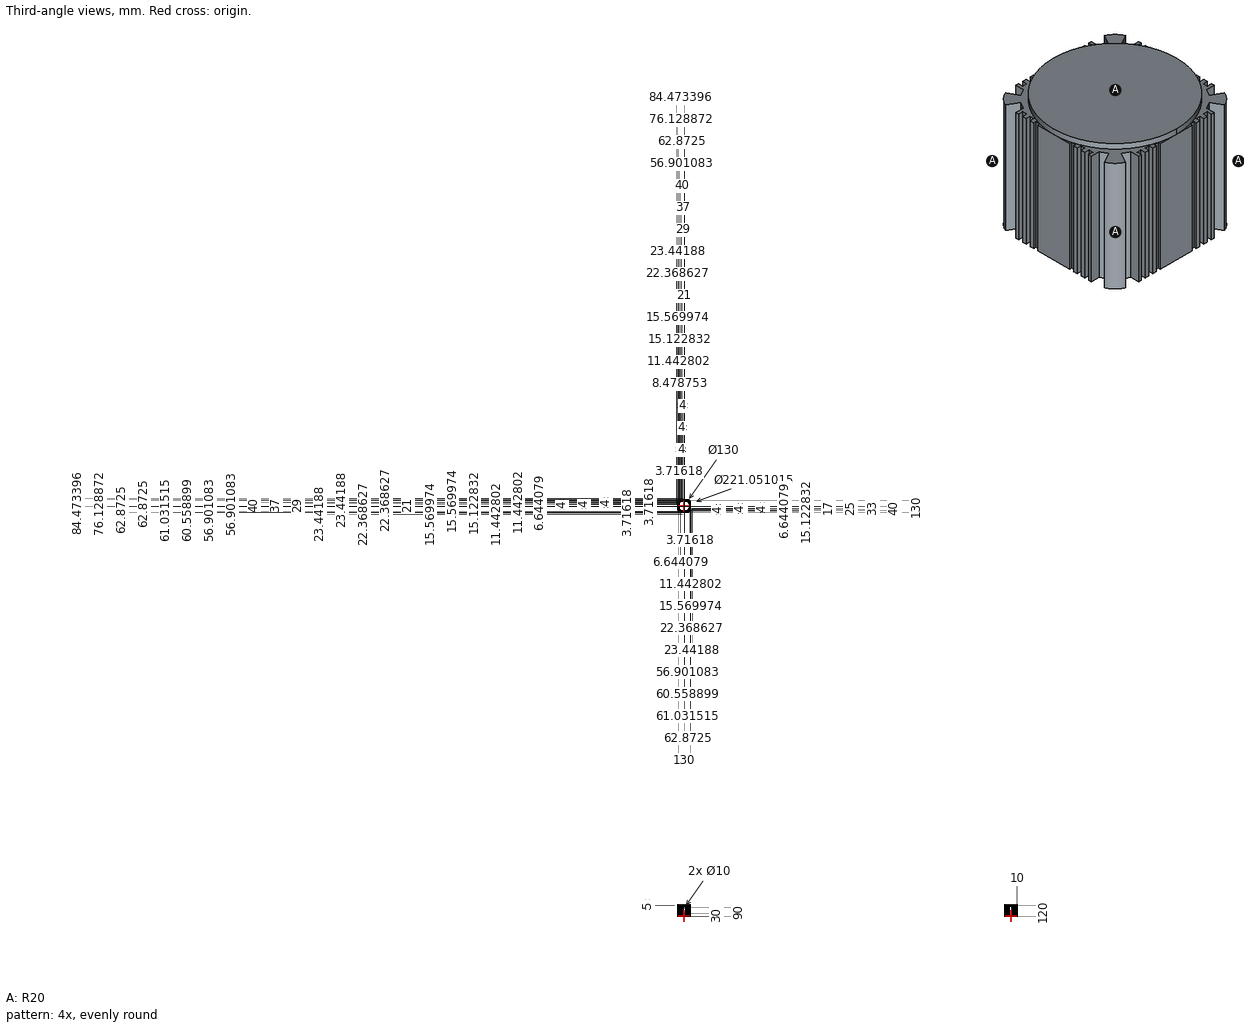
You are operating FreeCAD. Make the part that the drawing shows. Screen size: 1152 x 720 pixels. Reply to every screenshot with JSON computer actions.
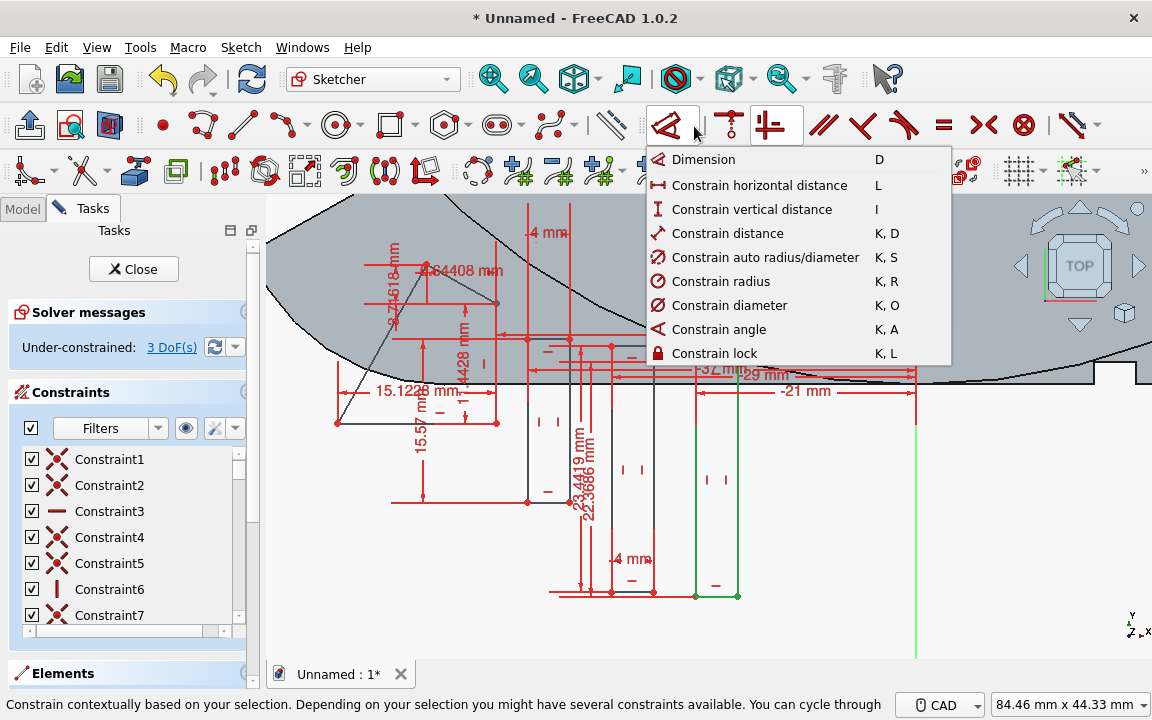
{"action": "left_click", "coordinate": [799, 209]}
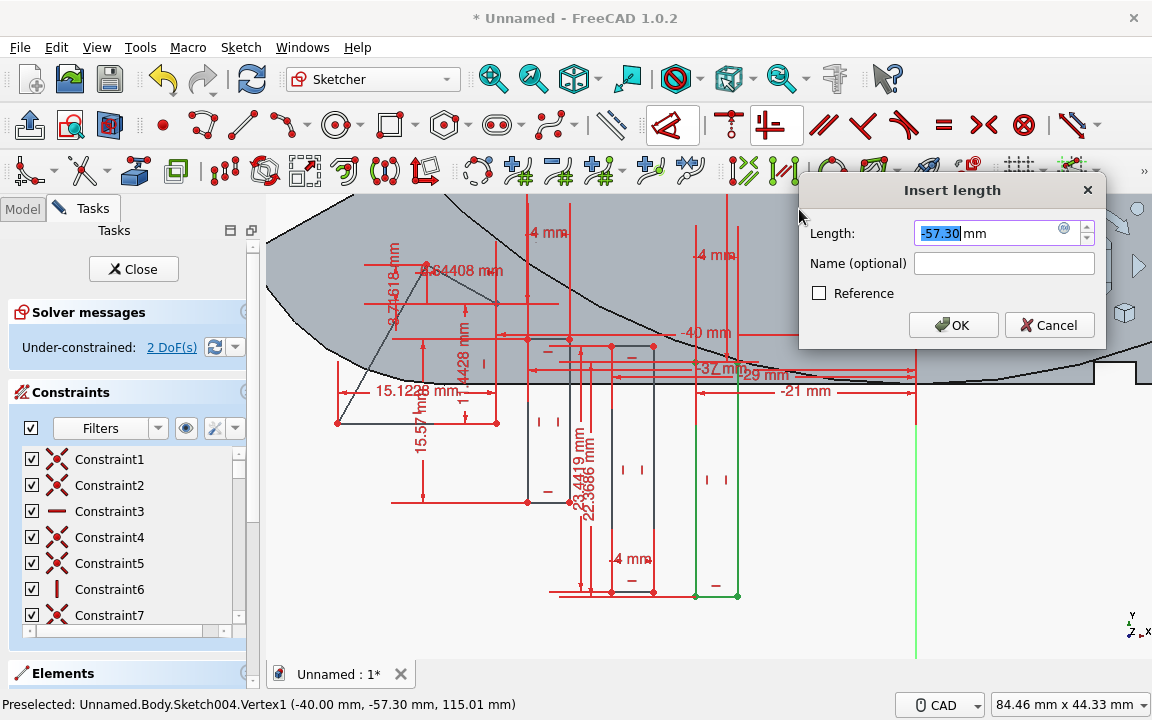
{"action": "type", "text": "-56.901083"}
{"action": "key", "text": "Return"}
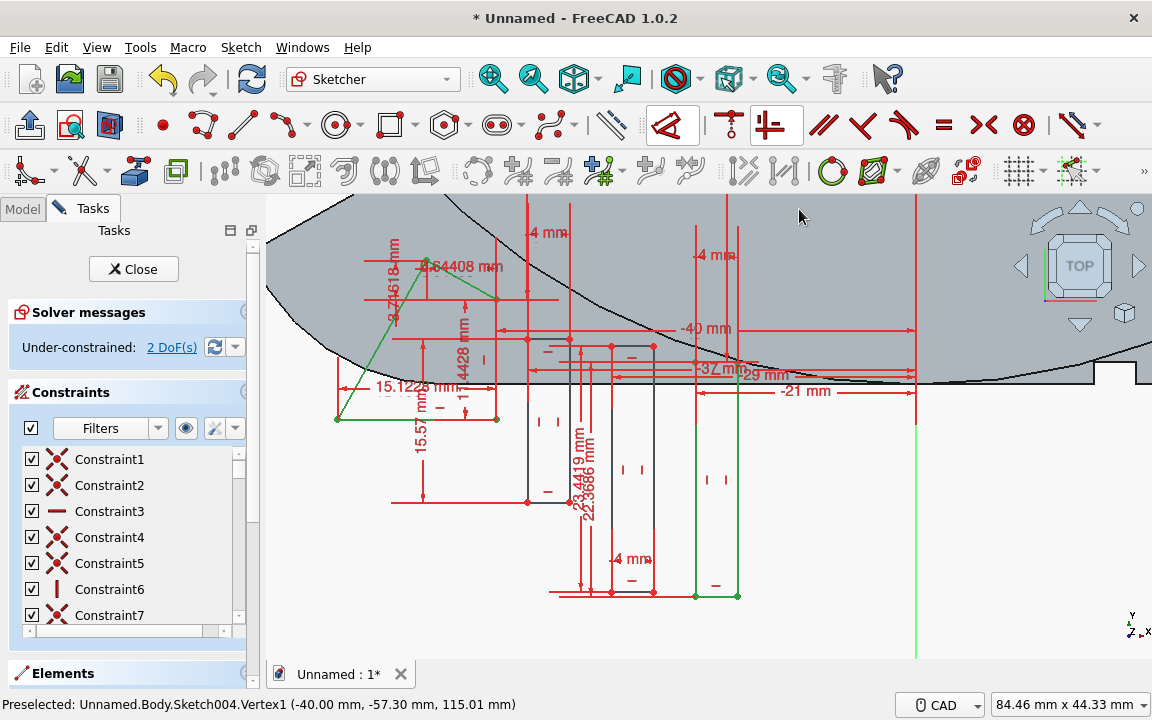
{"action": "left_click", "coordinate": [528, 339]}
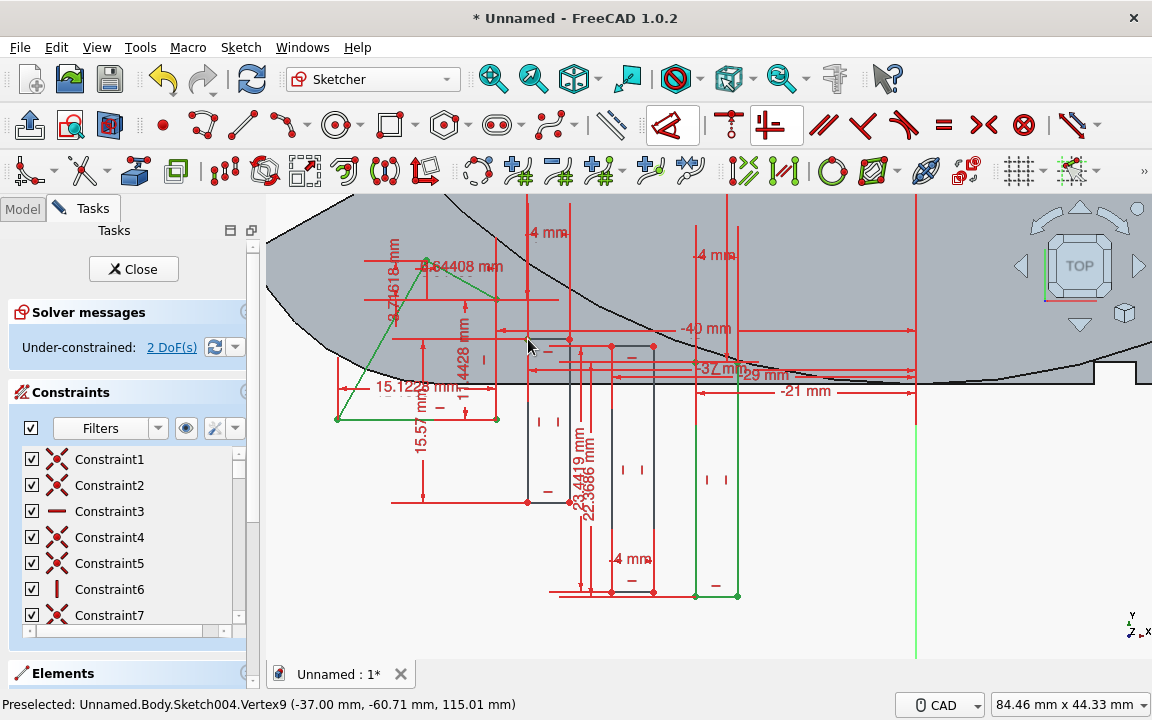
{"action": "left_click", "coordinate": [694, 126]}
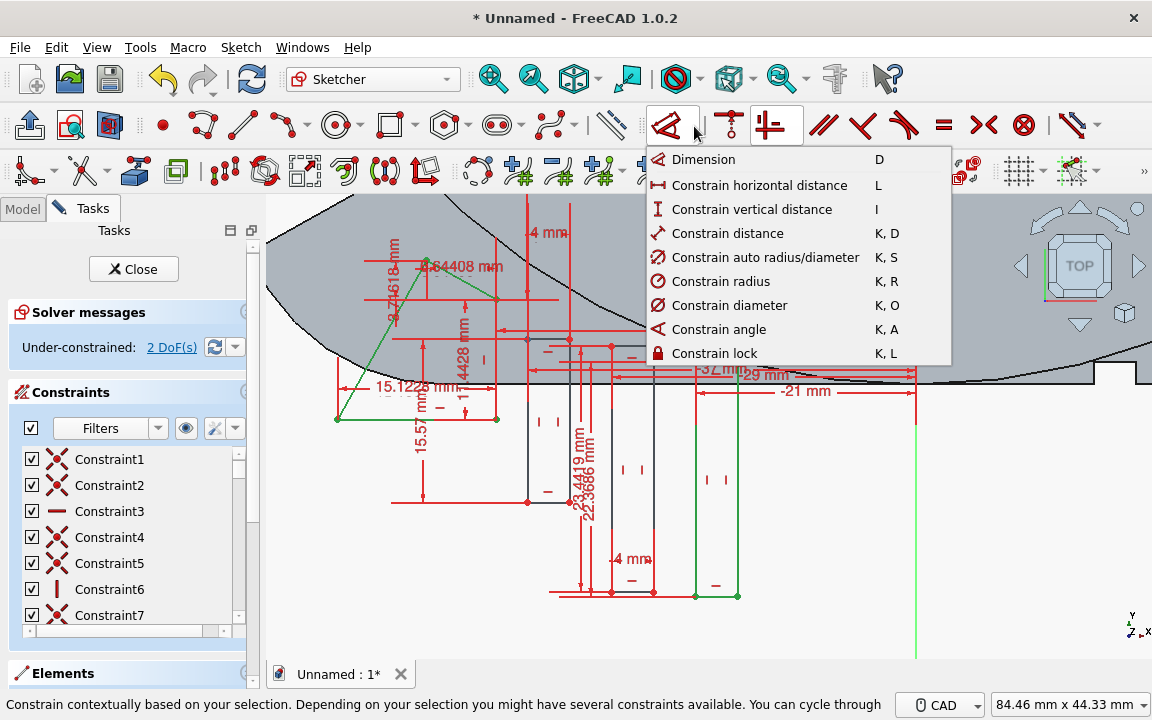
{"action": "left_click", "coordinate": [799, 209]}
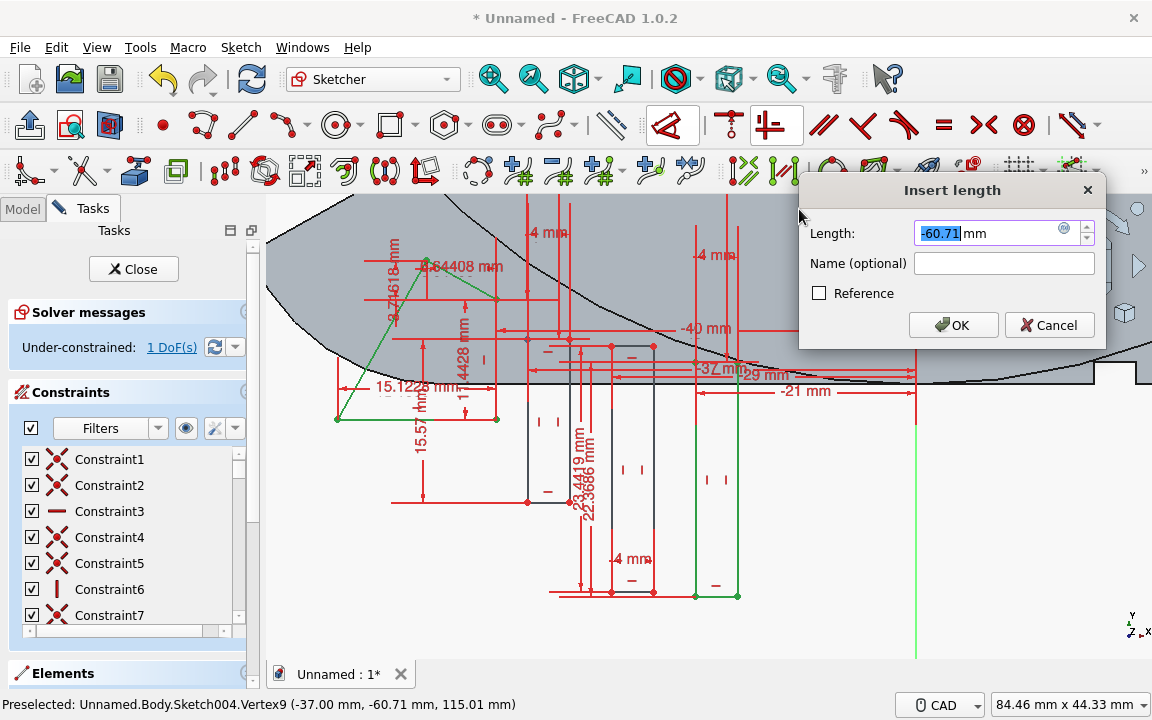
{"action": "type", "text": "-60.558899"}
{"action": "key", "text": "Return"}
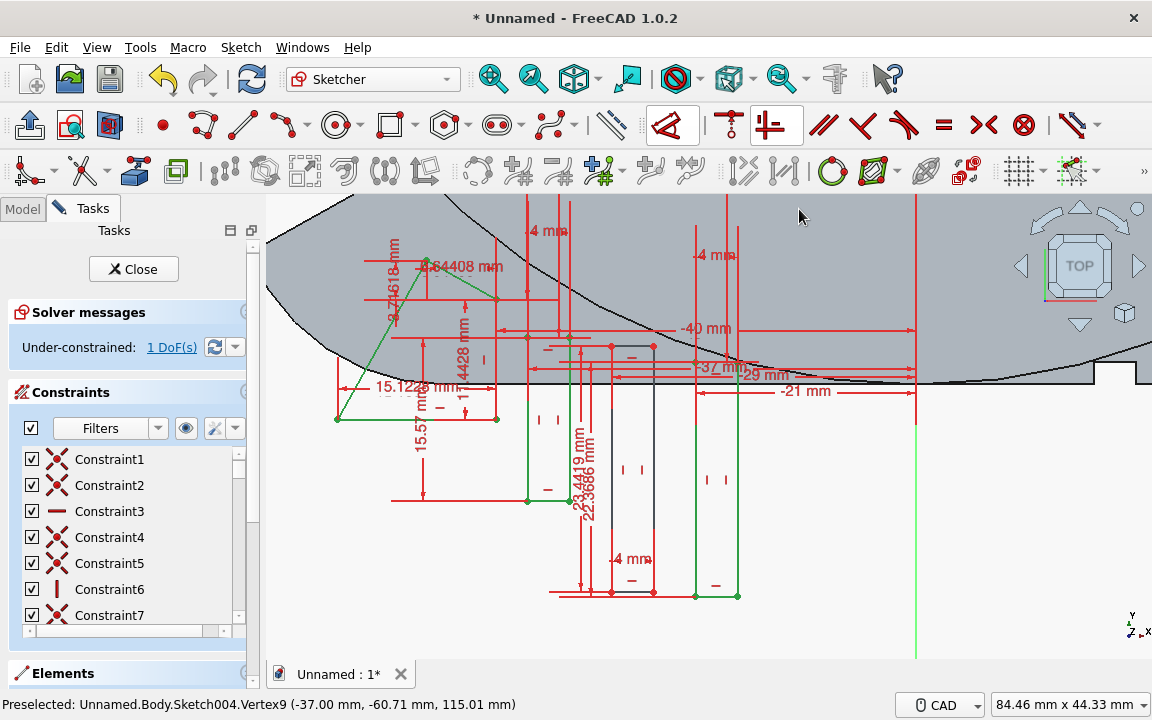
{"action": "left_click", "coordinate": [612, 346]}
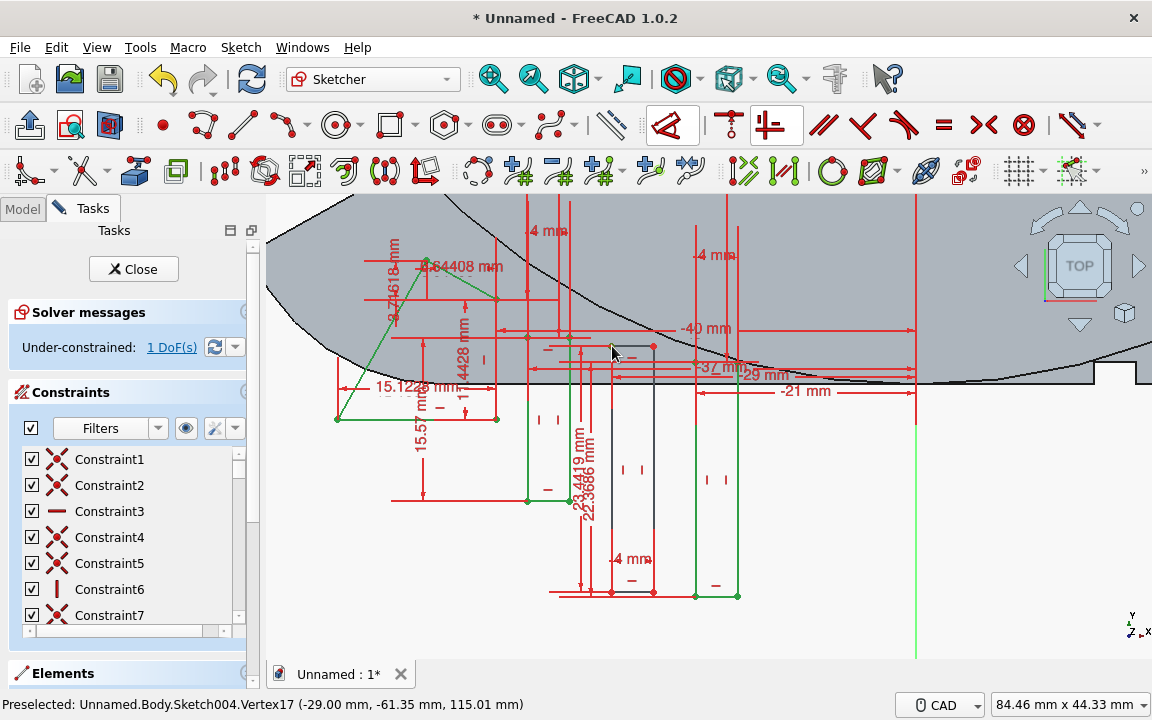
{"action": "left_click", "coordinate": [694, 126]}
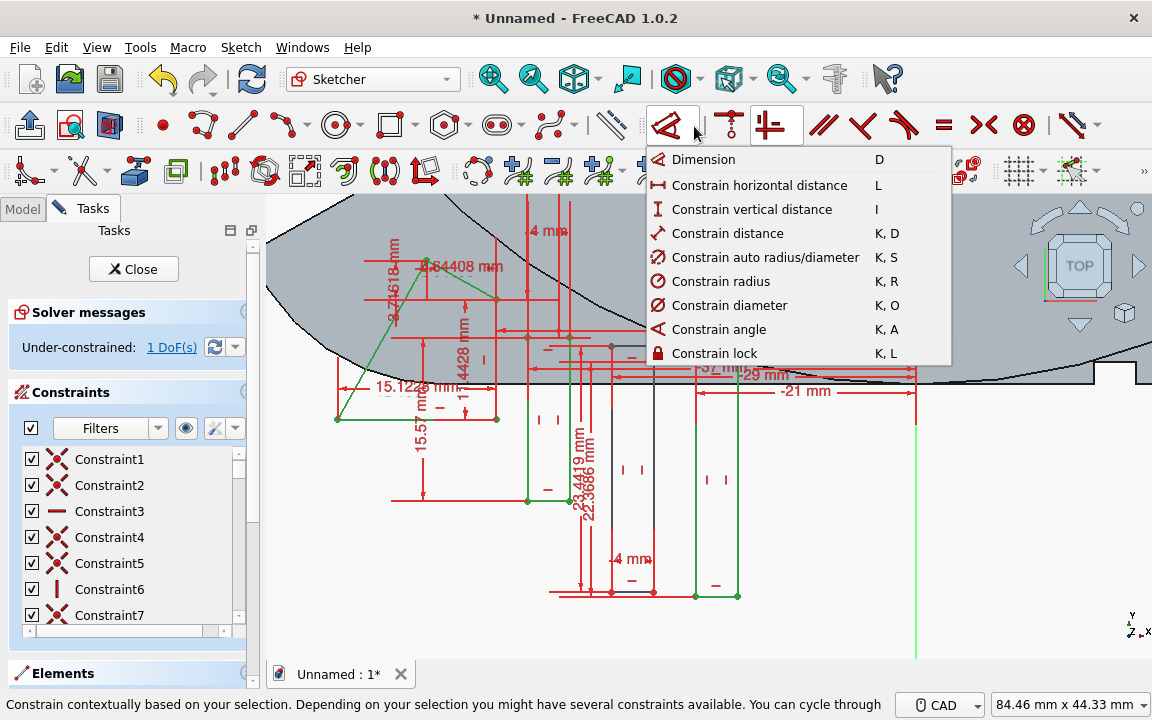
{"action": "left_click", "coordinate": [799, 209]}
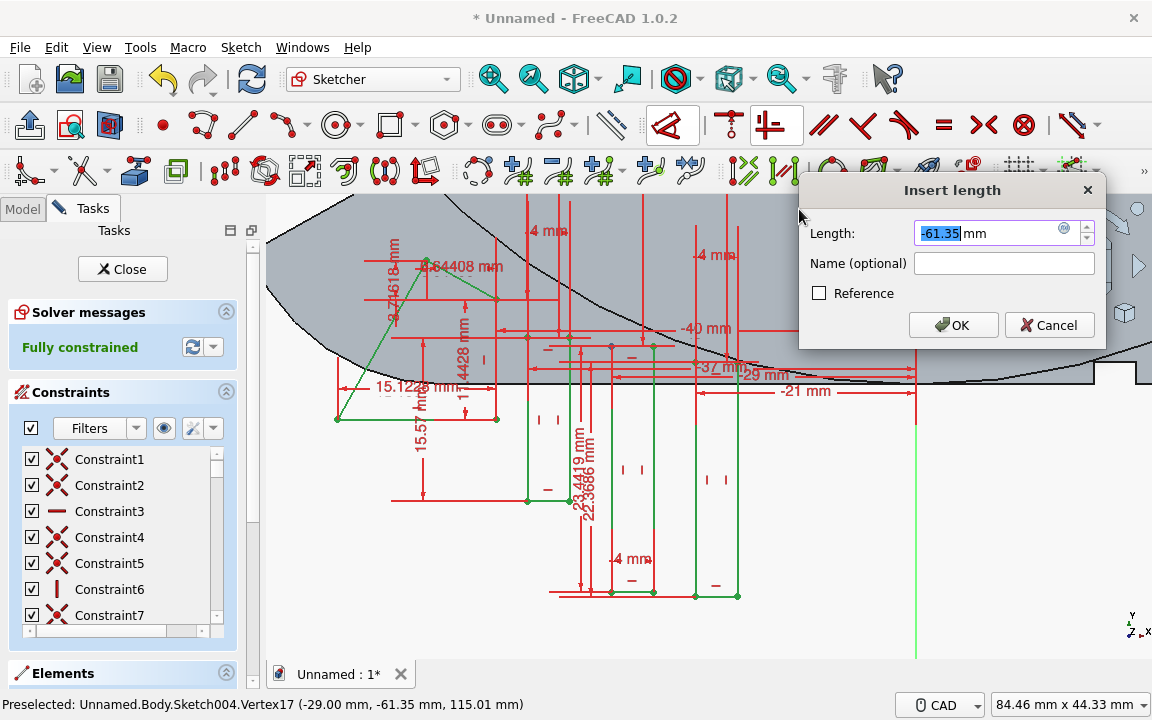
{"action": "type", "text": "-61.031515"}
{"action": "key", "text": "Return"}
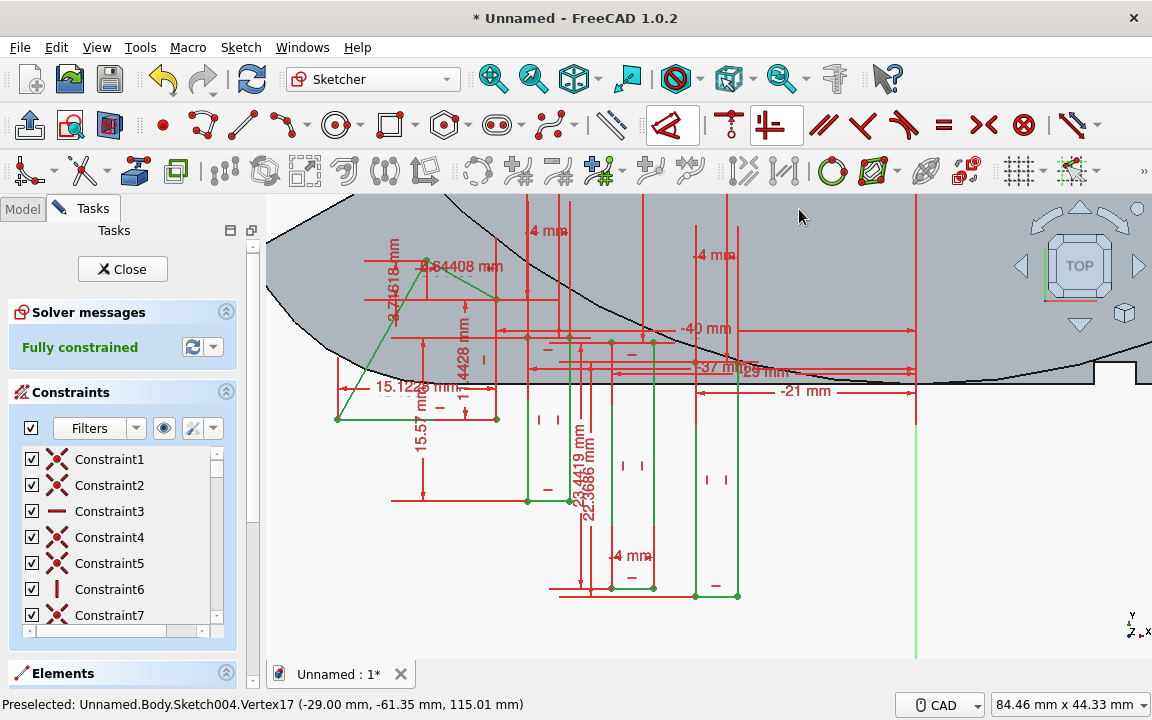
{"action": "left_click", "coordinate": [123, 269]}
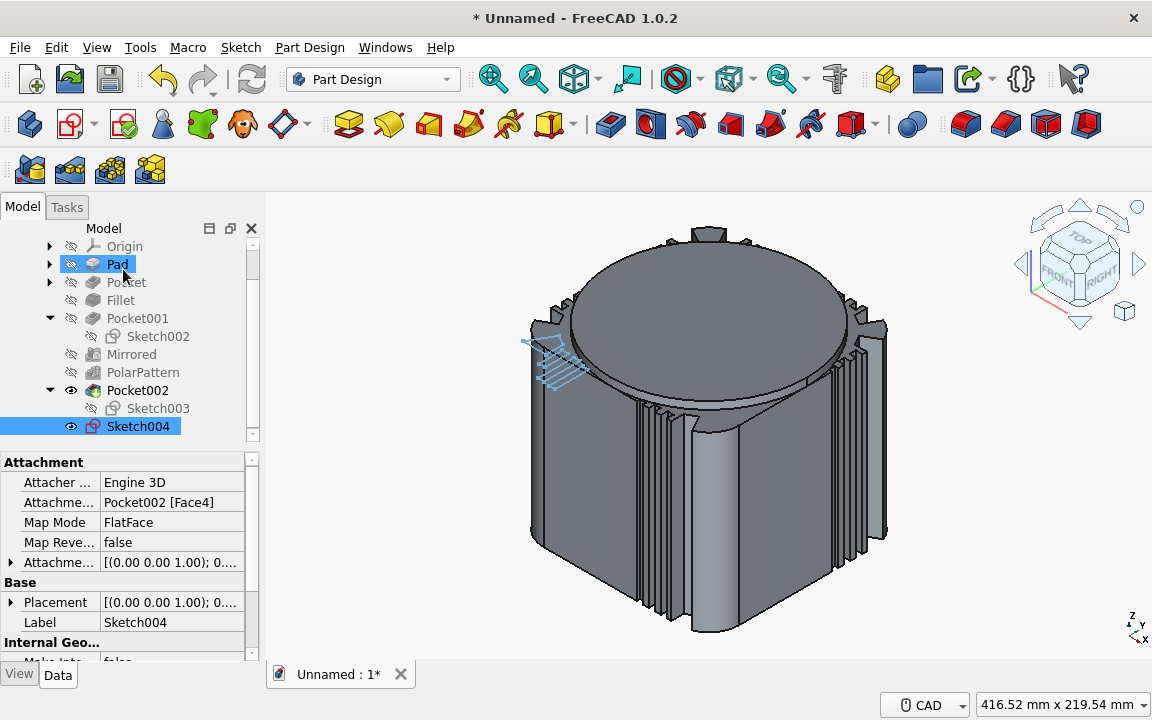
{"action": "left_click", "coordinate": [612, 124]}